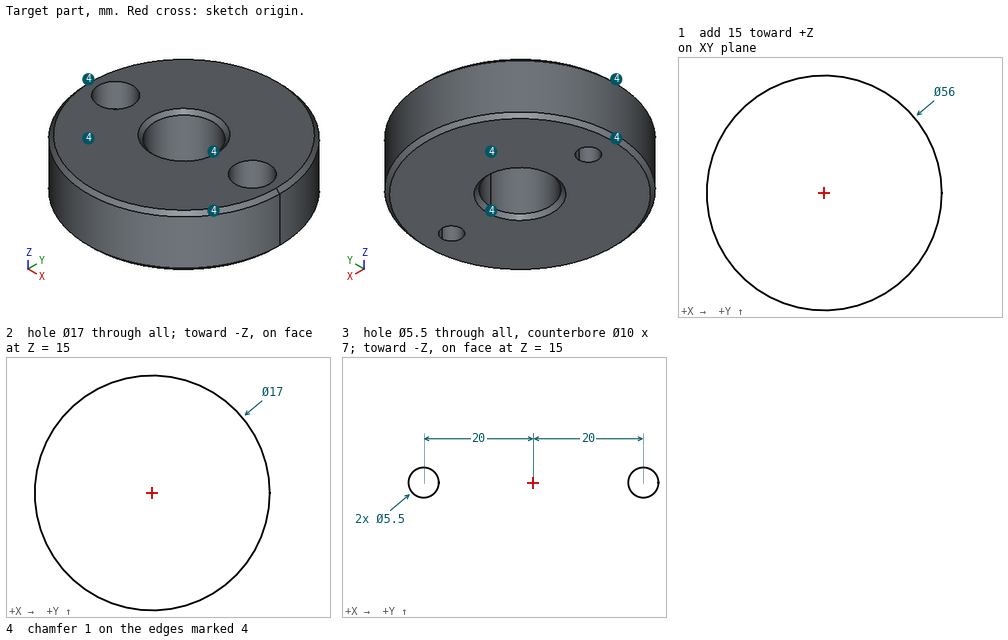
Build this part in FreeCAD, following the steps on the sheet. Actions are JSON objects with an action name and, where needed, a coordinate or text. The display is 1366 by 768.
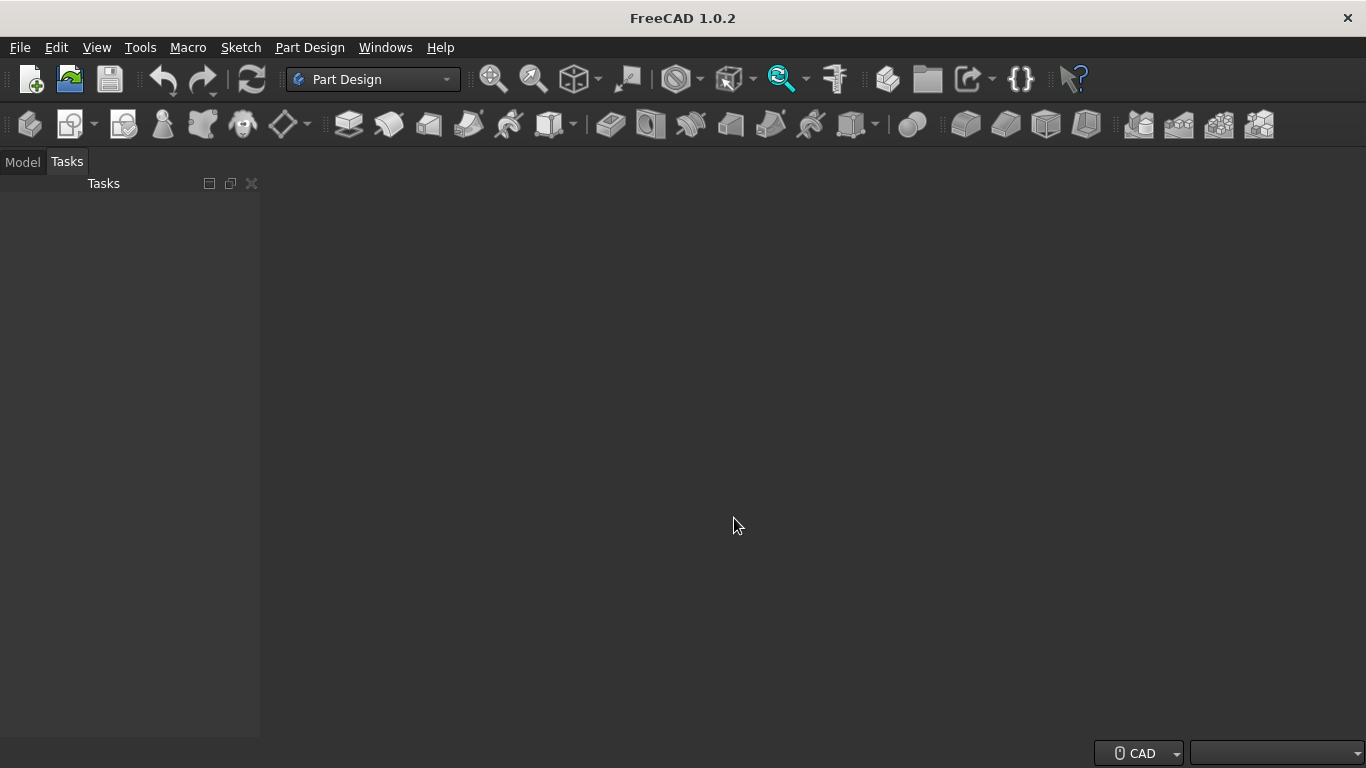
{"action": "key", "text": "ctrl+n"}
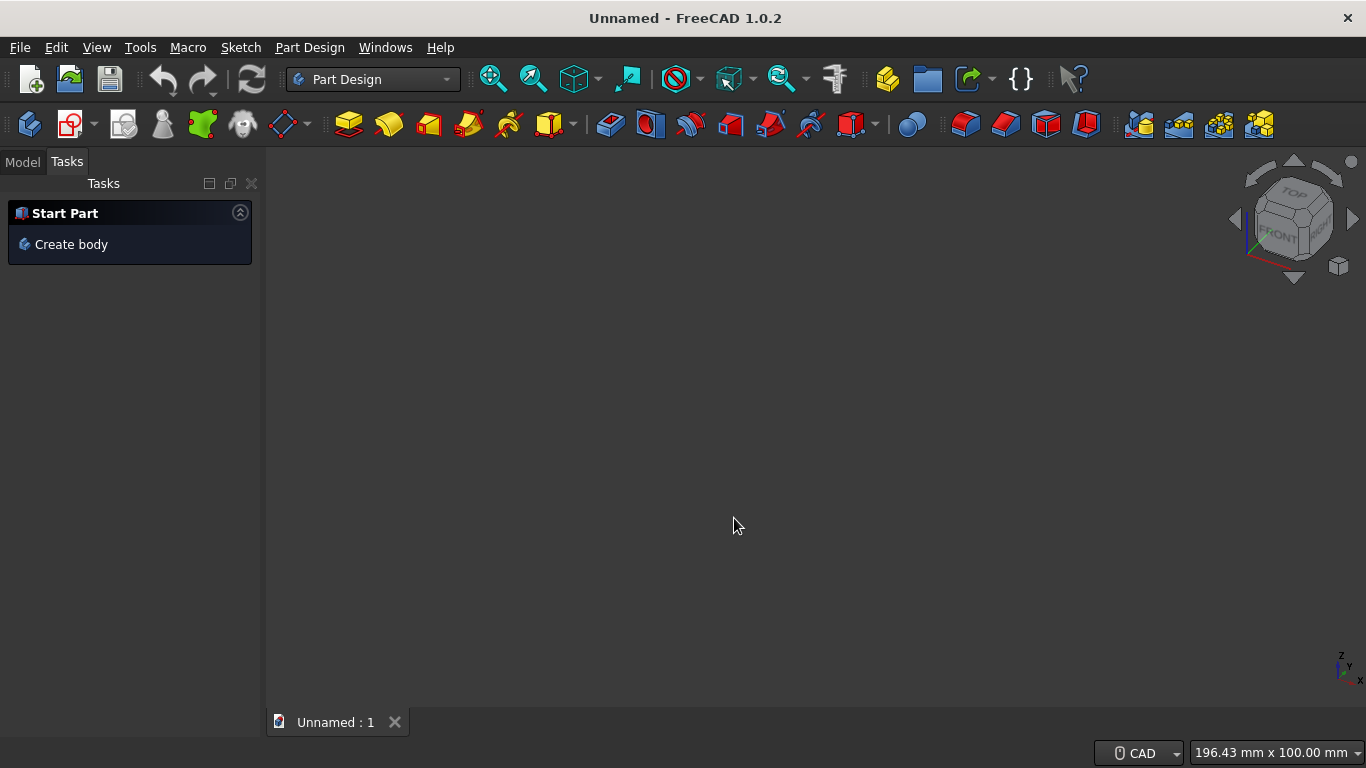
{"action": "left_click", "coordinate": [70, 124]}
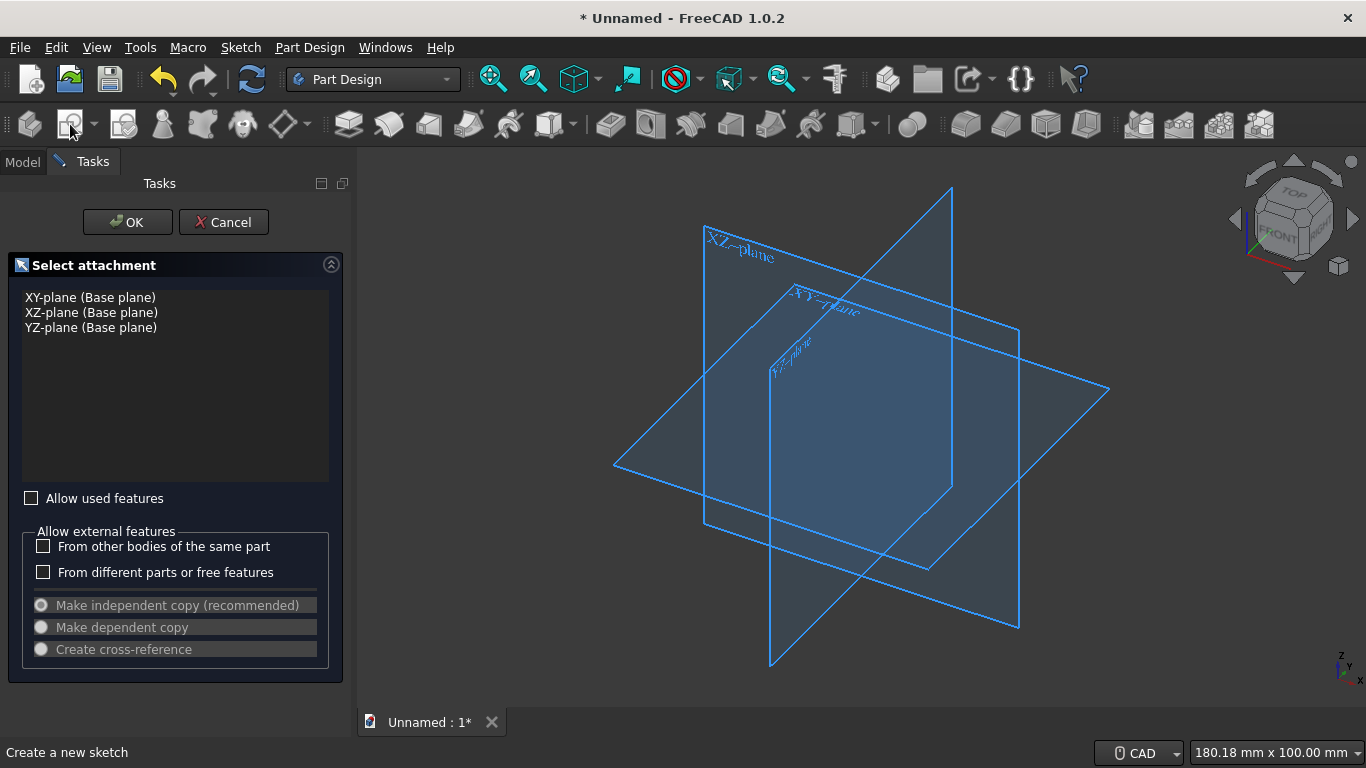
{"action": "left_click", "coordinate": [82, 298]}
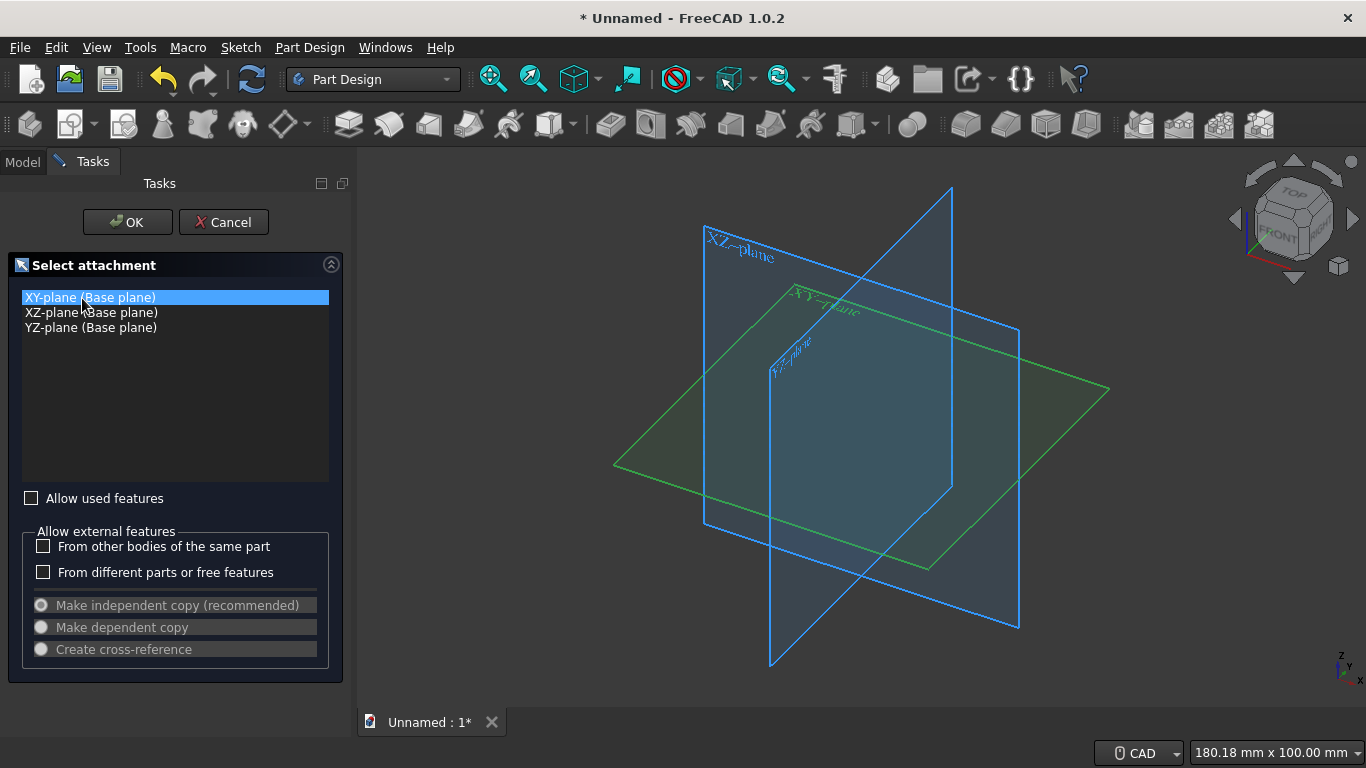
{"action": "left_click", "coordinate": [128, 222]}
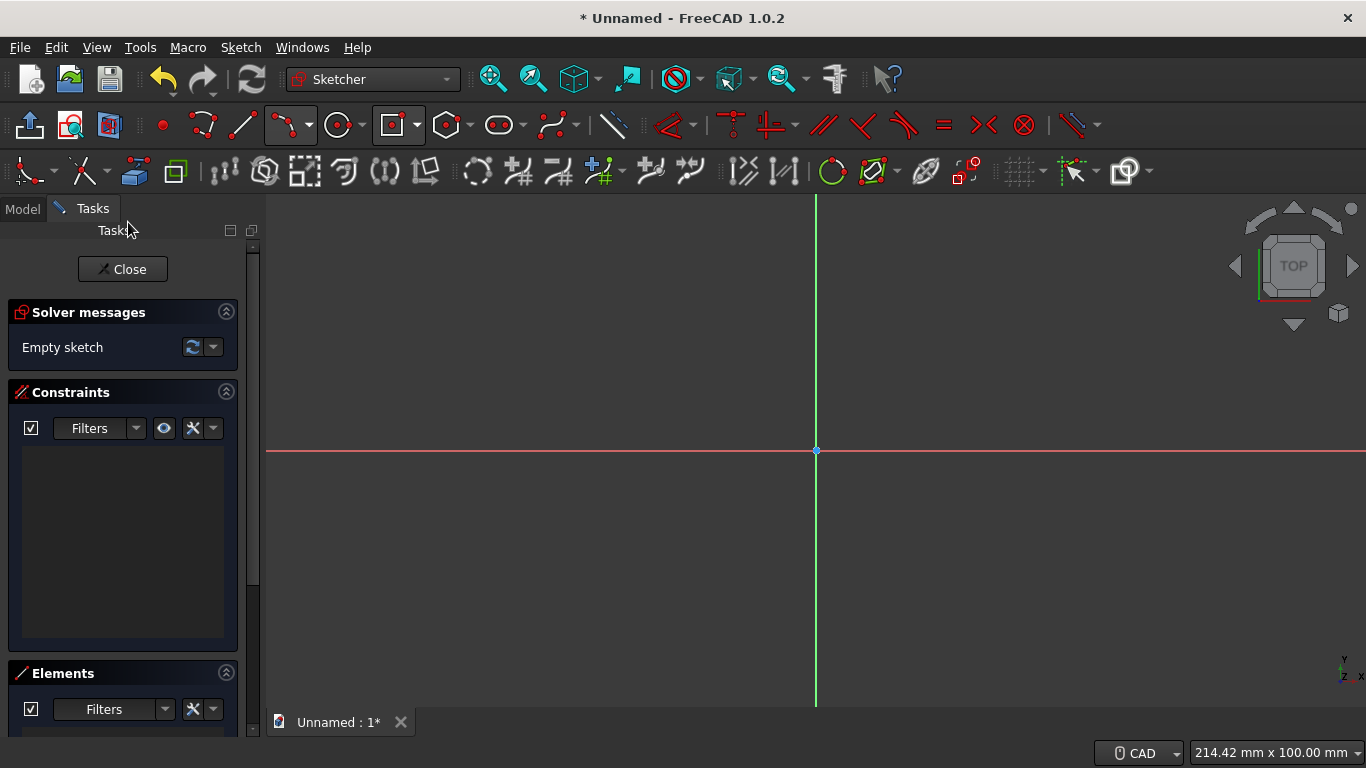
{"action": "left_click", "coordinate": [338, 126]}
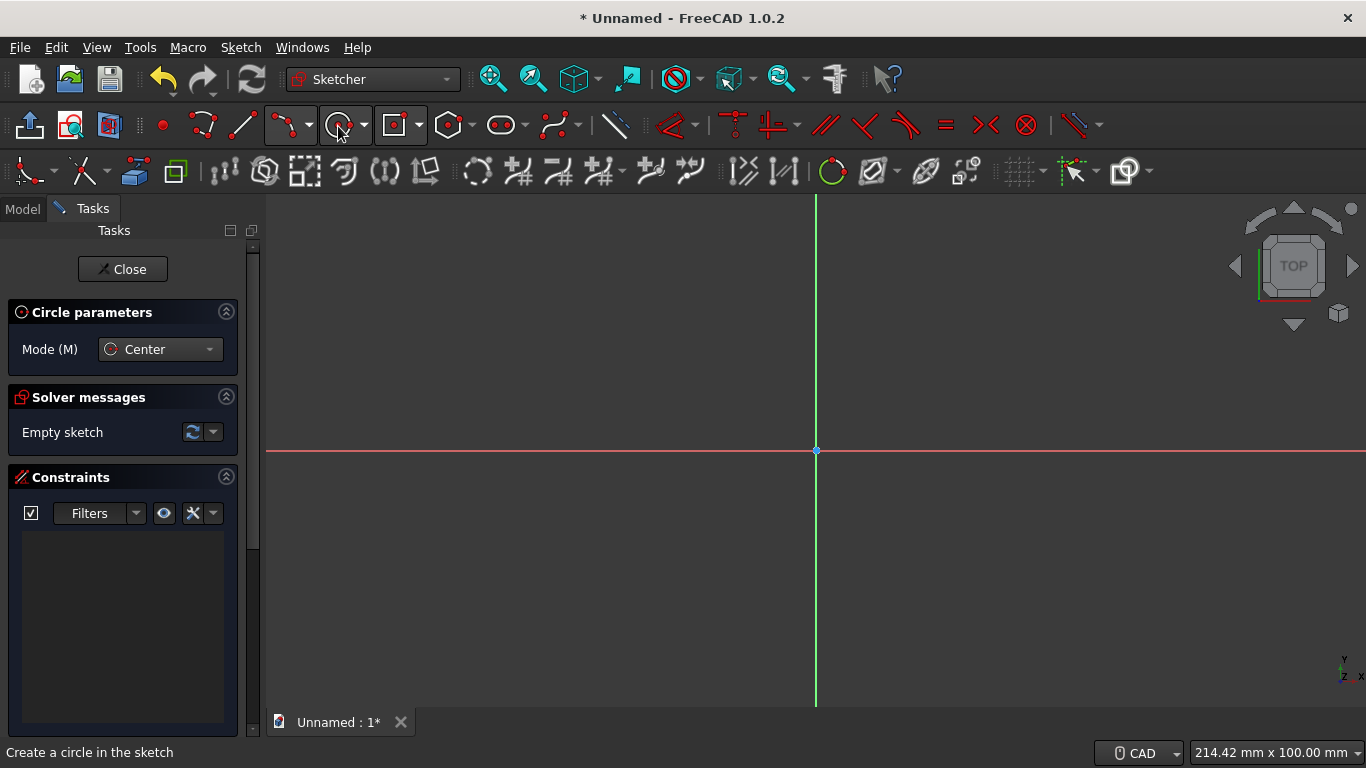
{"action": "left_click", "coordinate": [816, 450]}
{"action": "left_click", "coordinate": [918, 349]}
{"action": "key", "text": "Escape"}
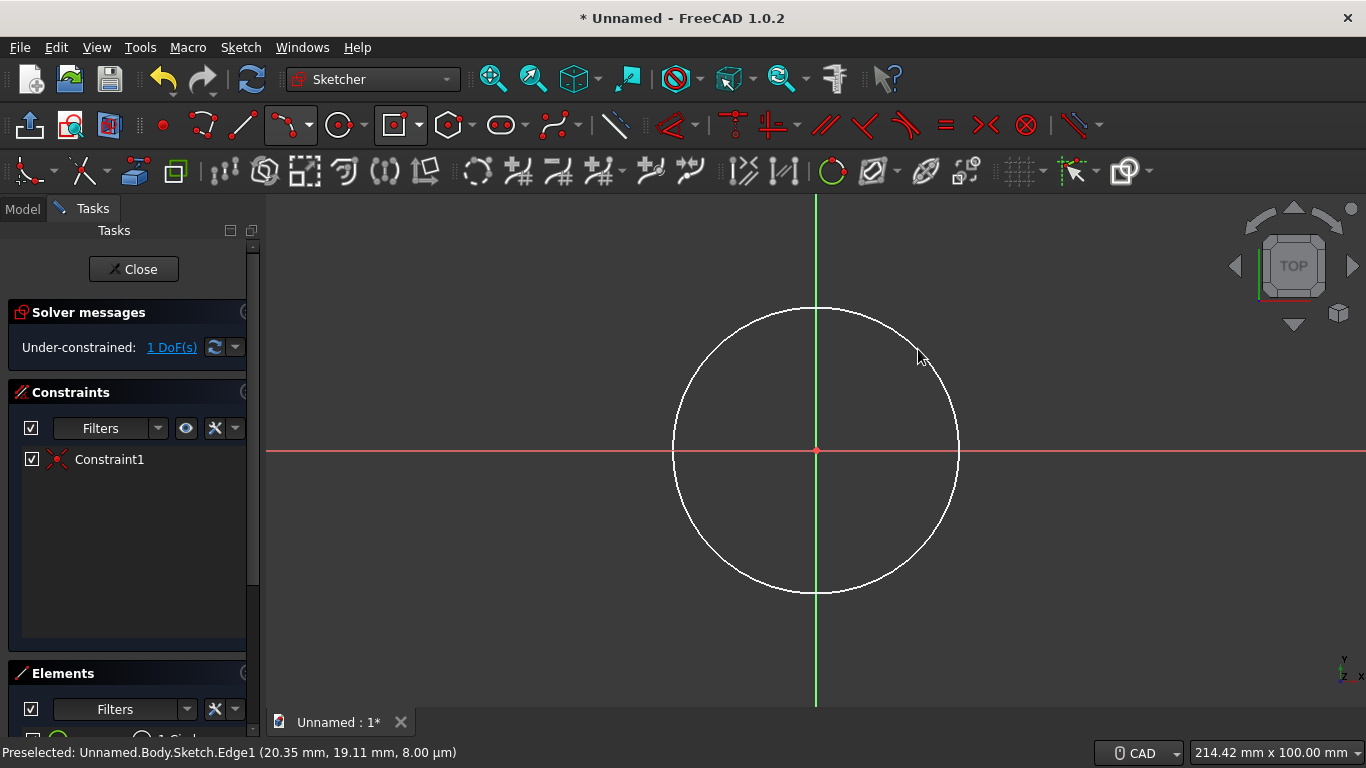
{"action": "key", "text": "d"}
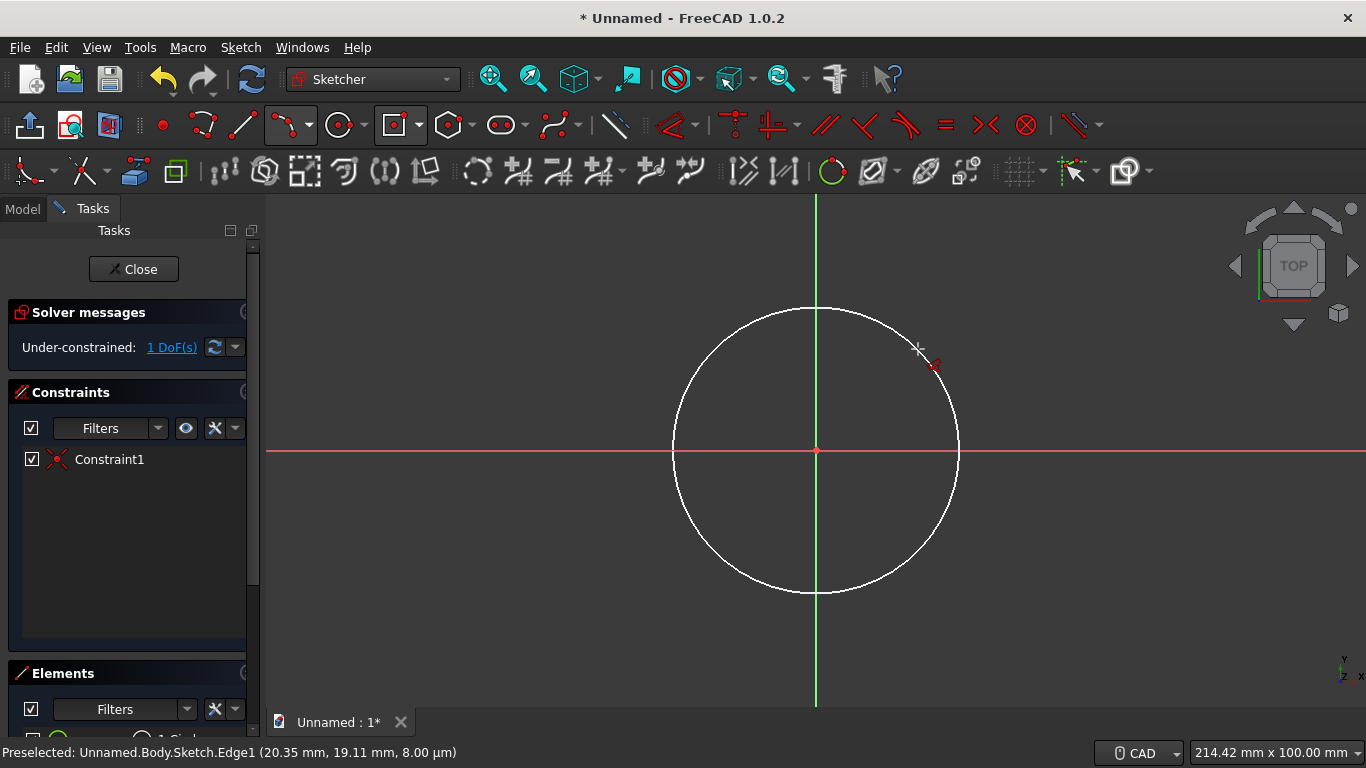
{"action": "left_click", "coordinate": [917, 349]}
{"action": "left_click", "coordinate": [940, 326]}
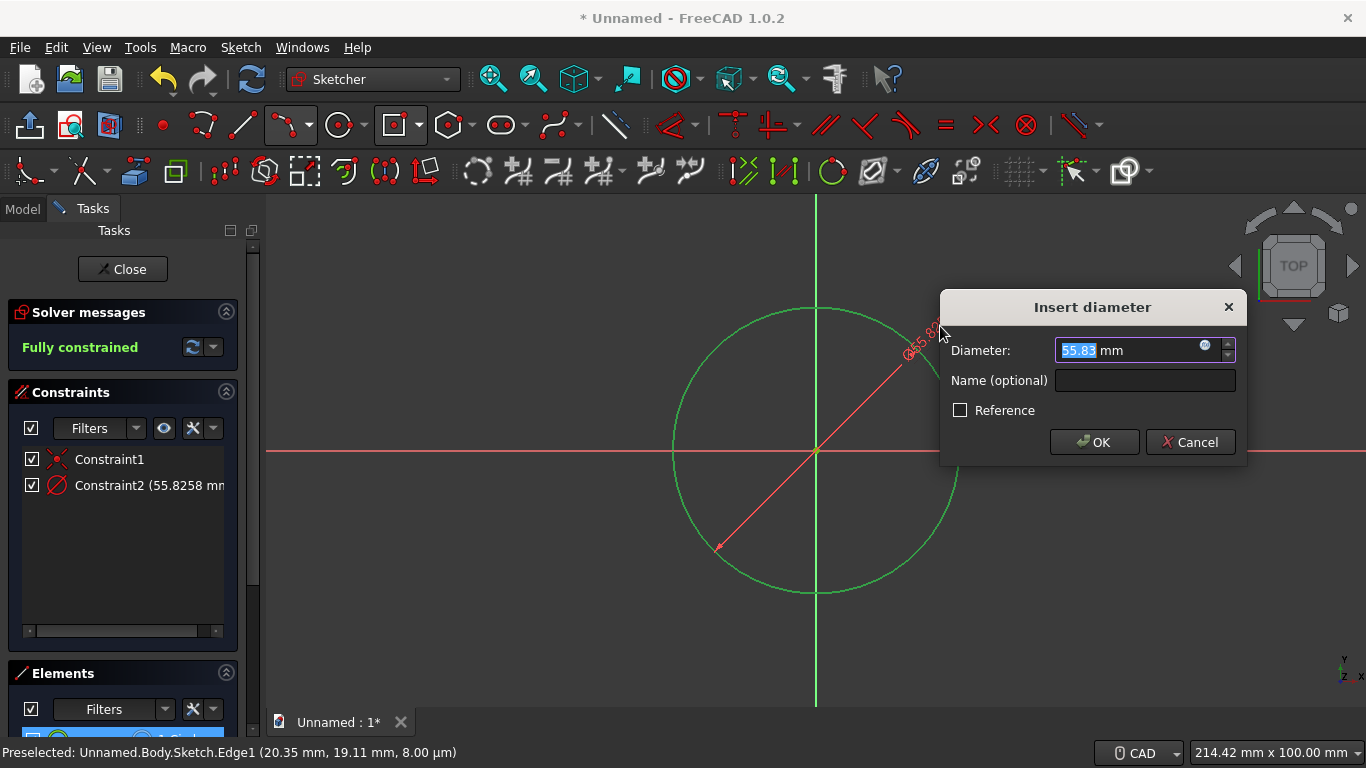
{"action": "type", "text": "56"}
{"action": "key", "text": "Return"}
{"action": "key", "text": "Escape"}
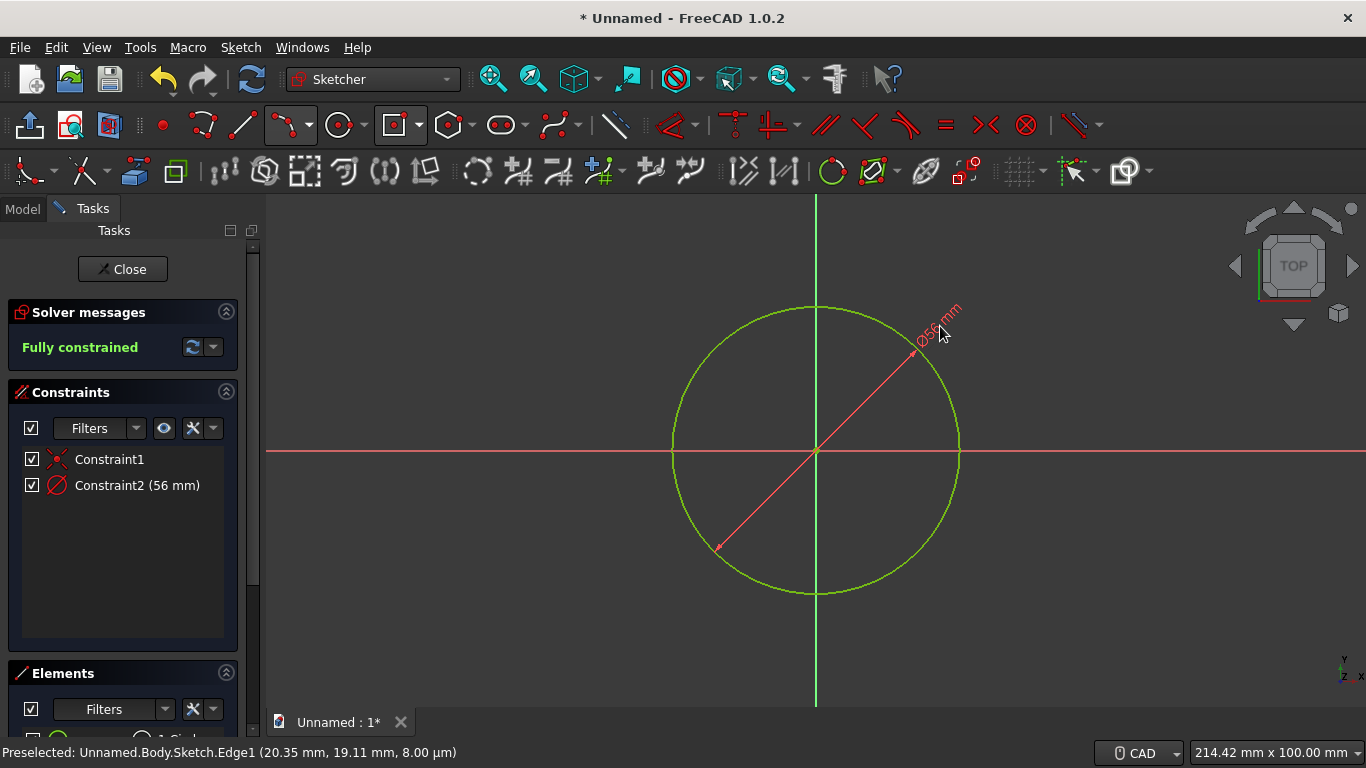
{"action": "left_click", "coordinate": [123, 269]}